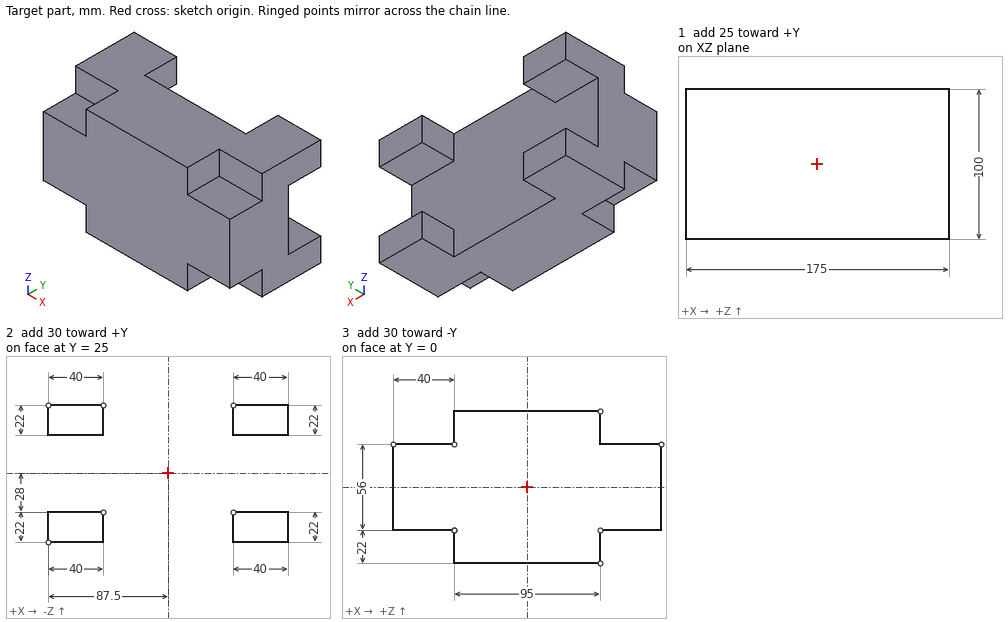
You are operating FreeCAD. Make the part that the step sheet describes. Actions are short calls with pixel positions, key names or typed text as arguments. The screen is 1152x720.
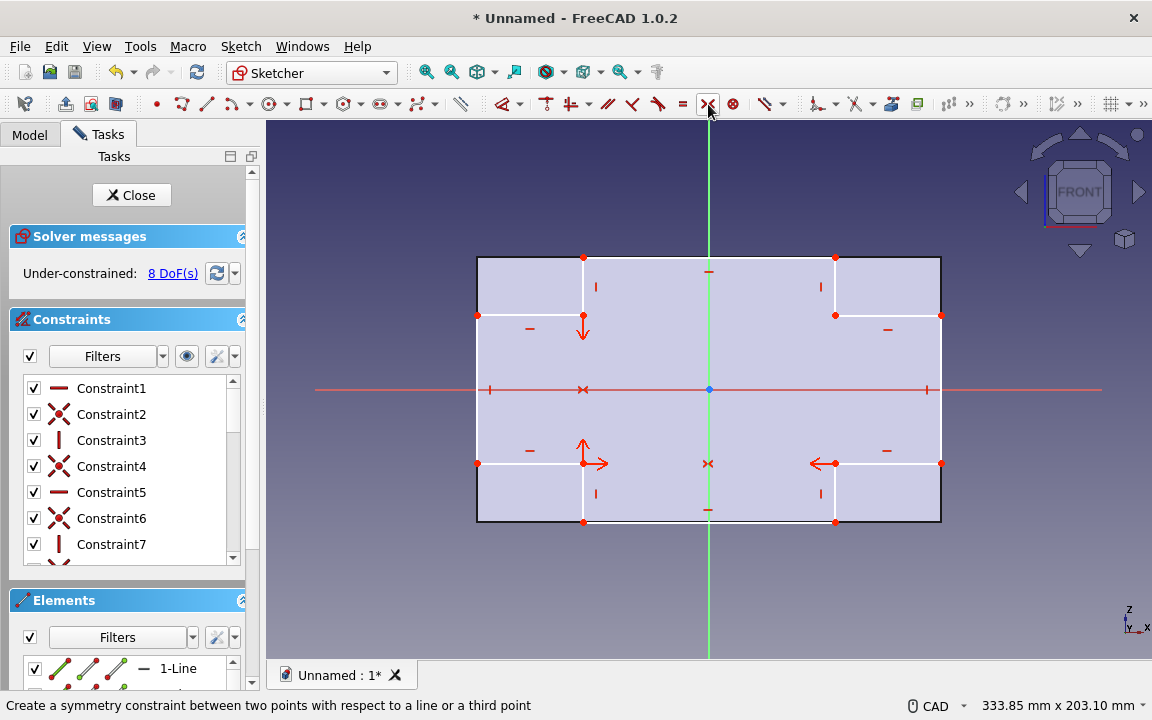
click(477, 315)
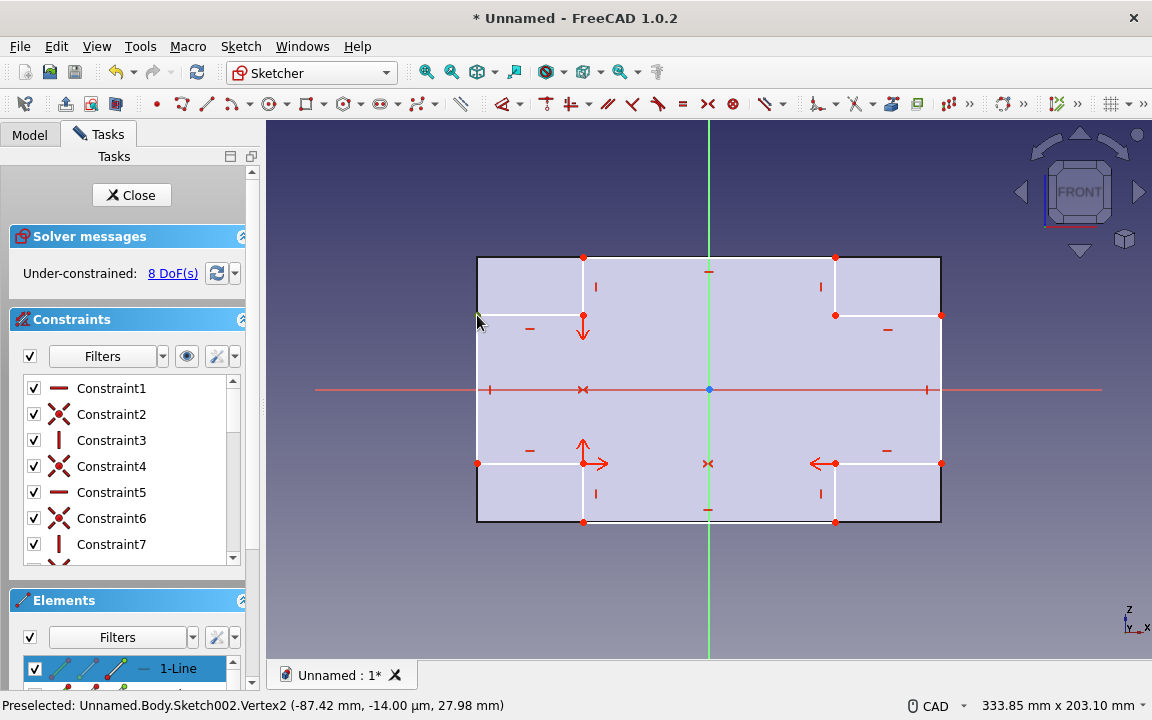
click(941, 316)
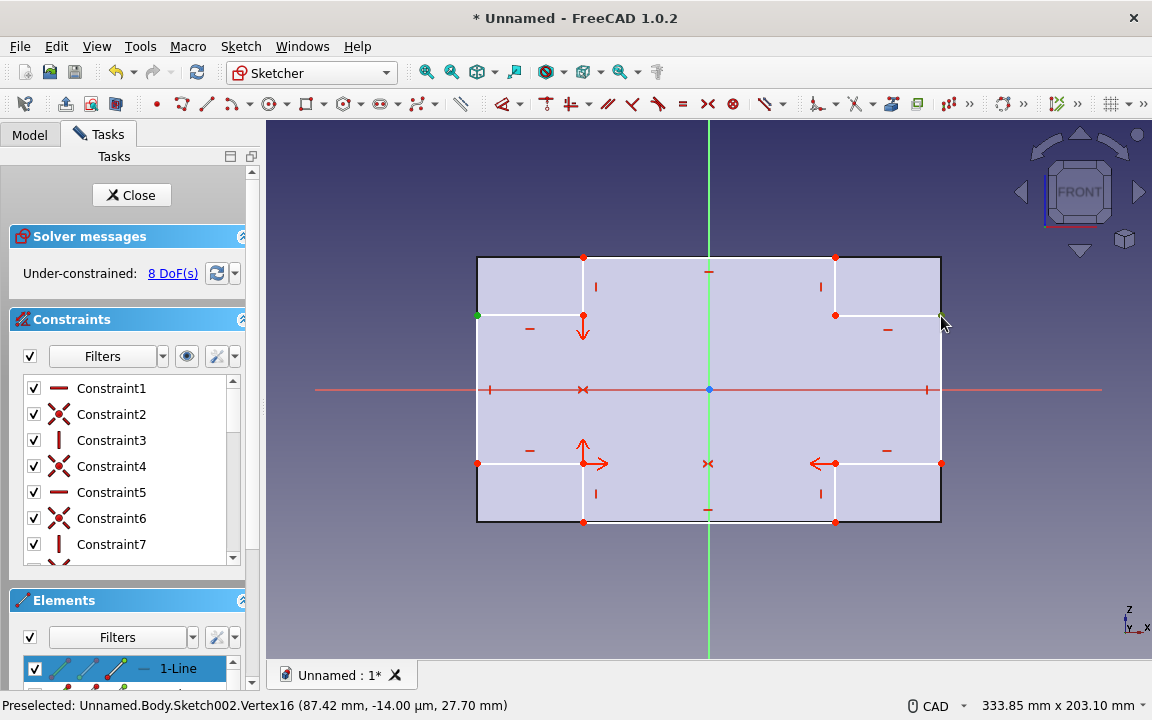
click(709, 596)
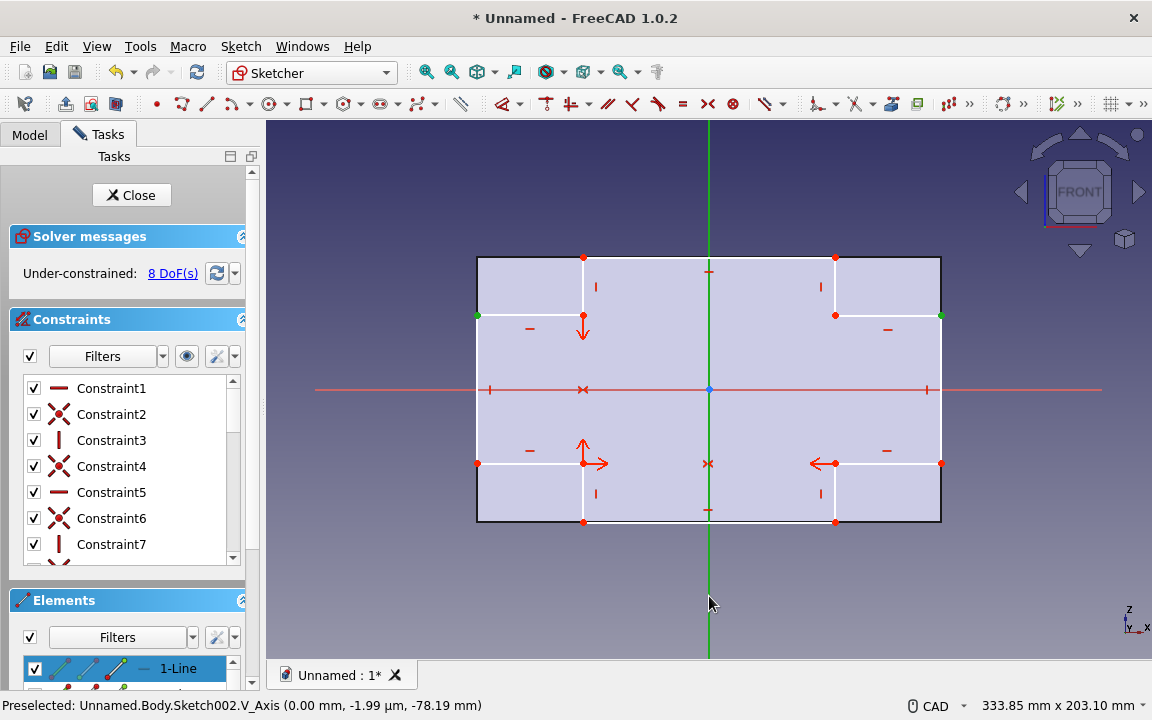
key(s)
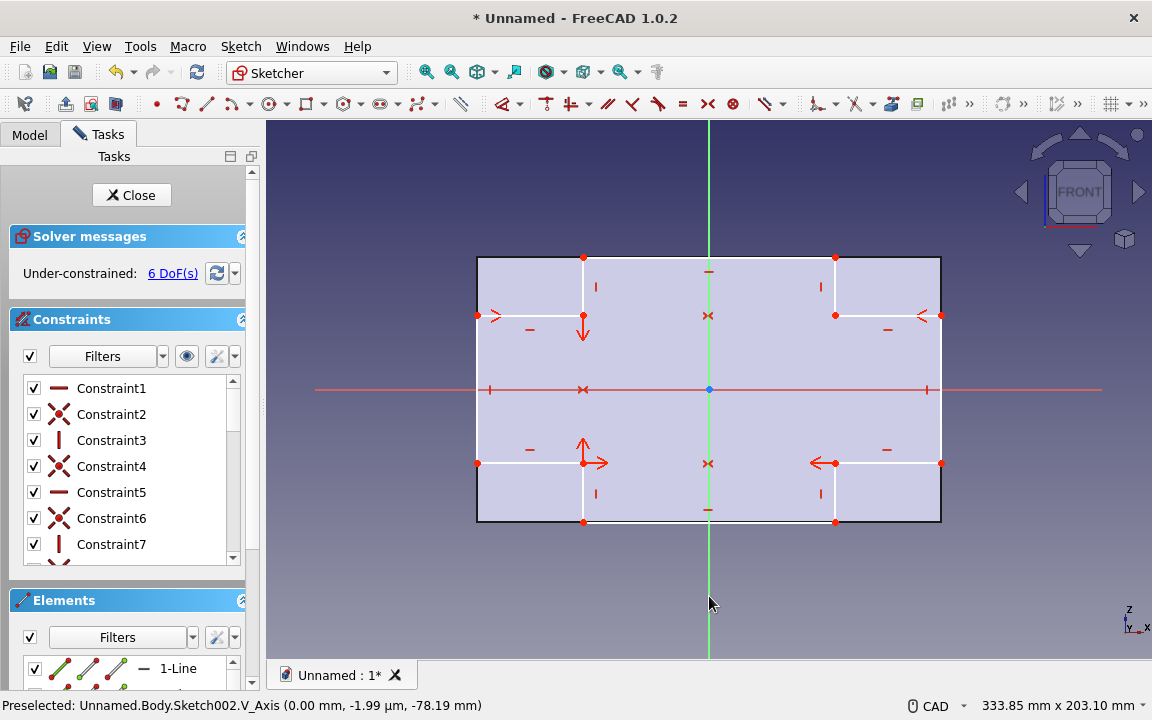
click(835, 523)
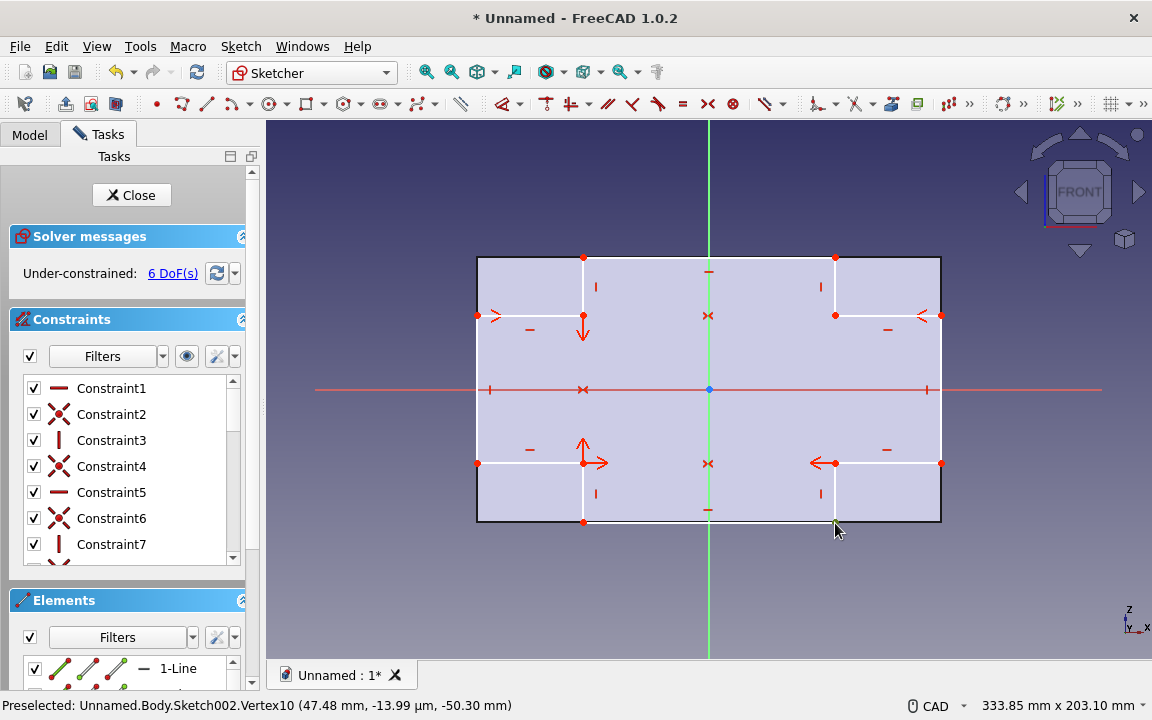
click(835, 258)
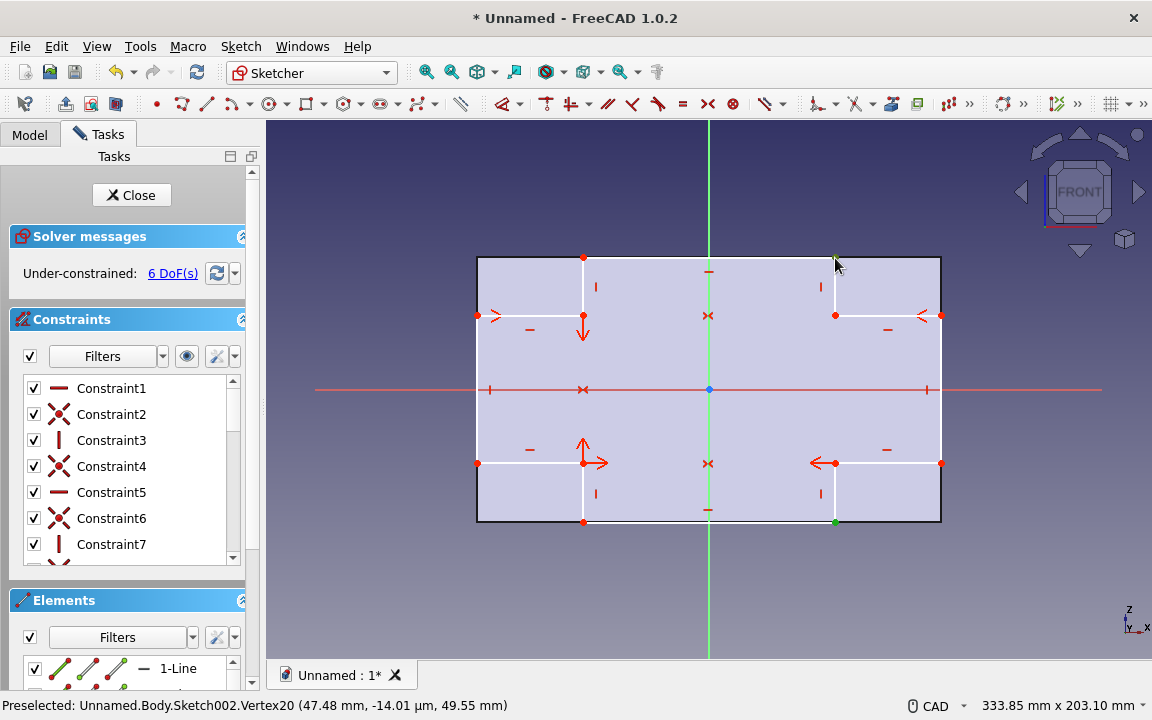
click(344, 390)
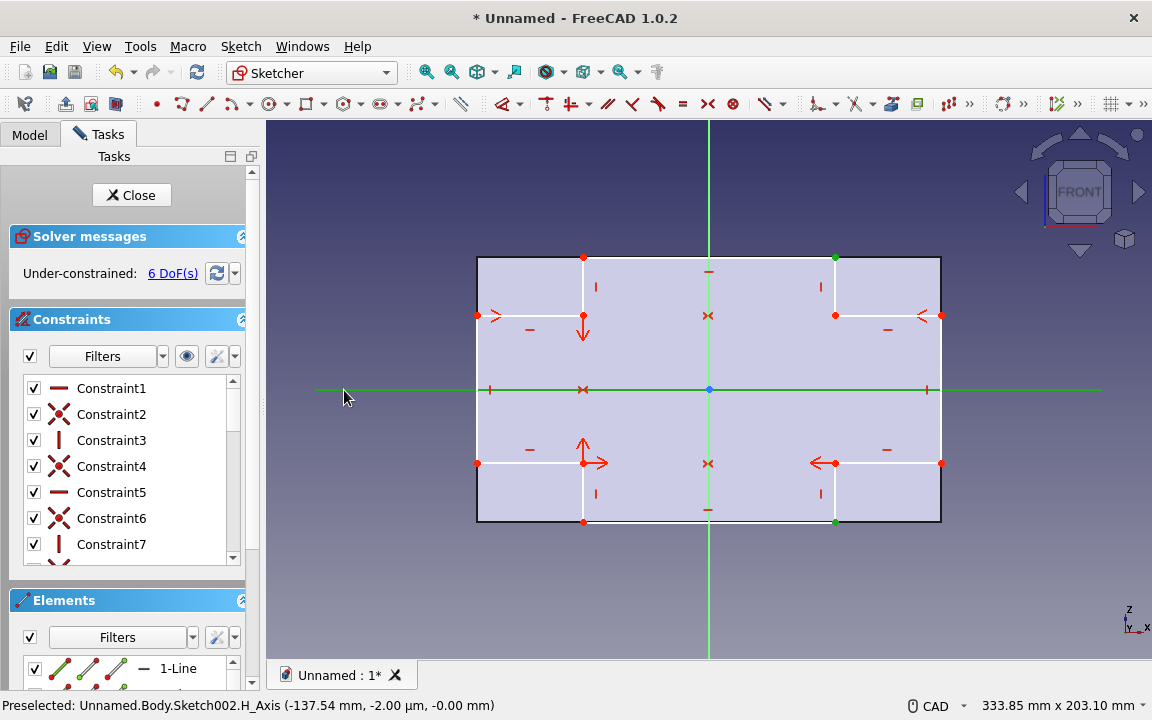
click(708, 104)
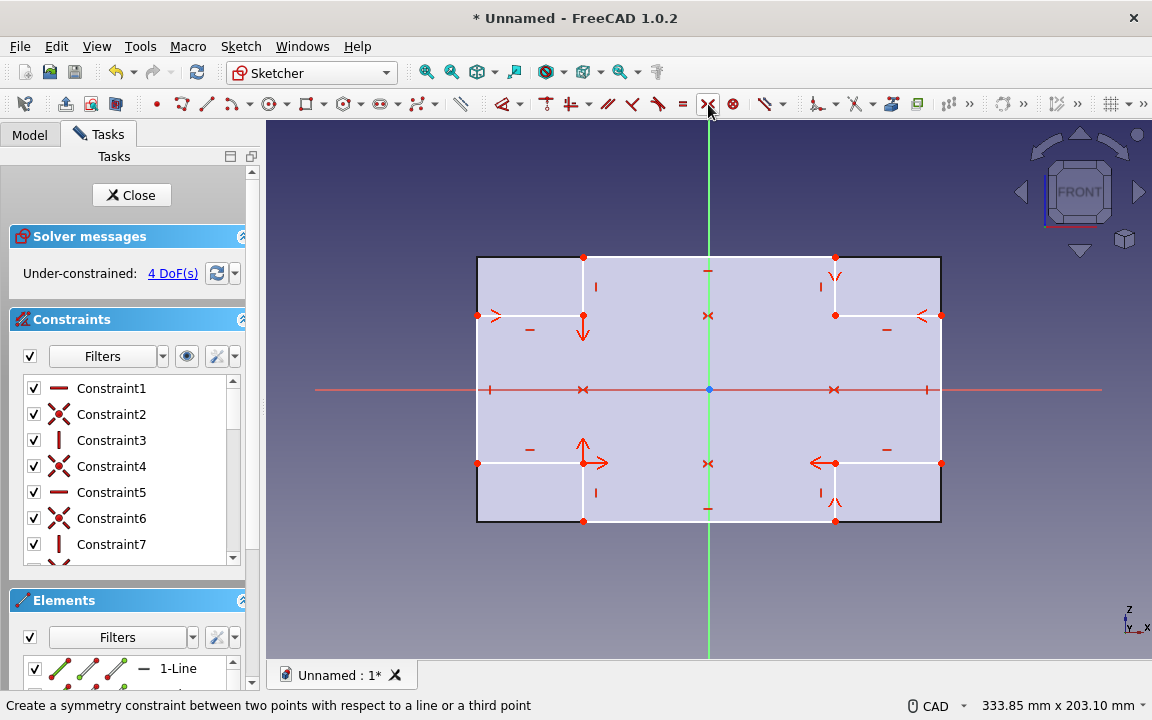
click(502, 104)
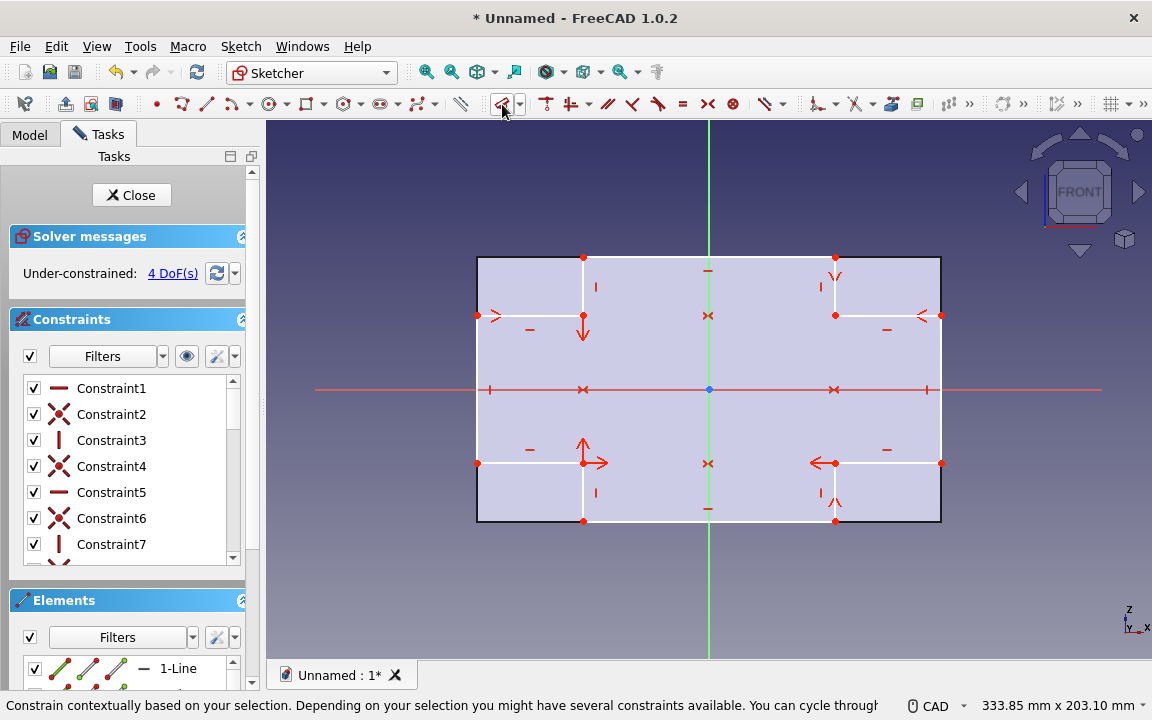
click(551, 316)
click(530, 282)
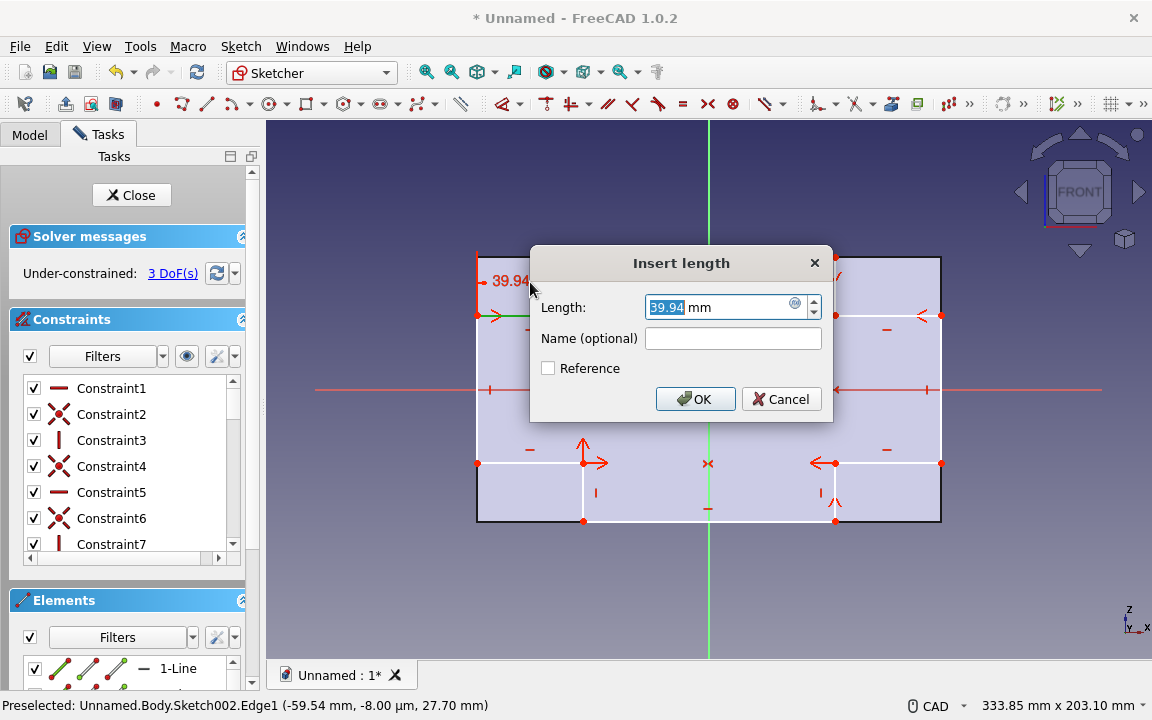
text(40)
key(Return)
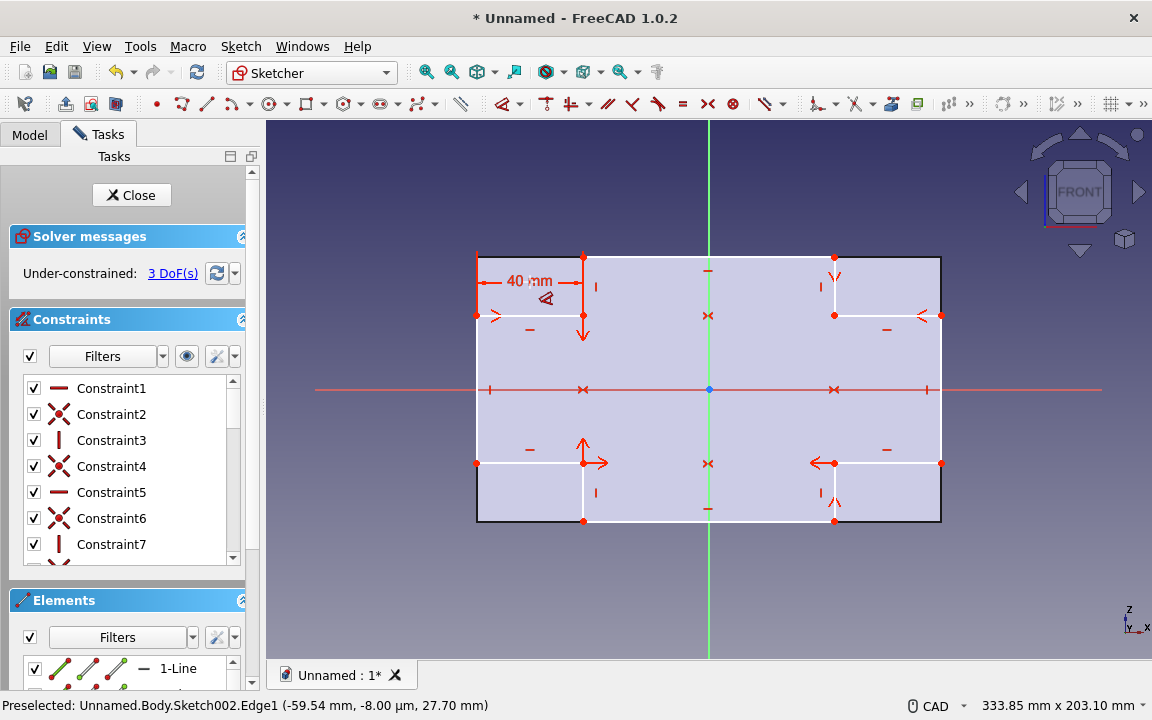
click(477, 360)
click(443, 356)